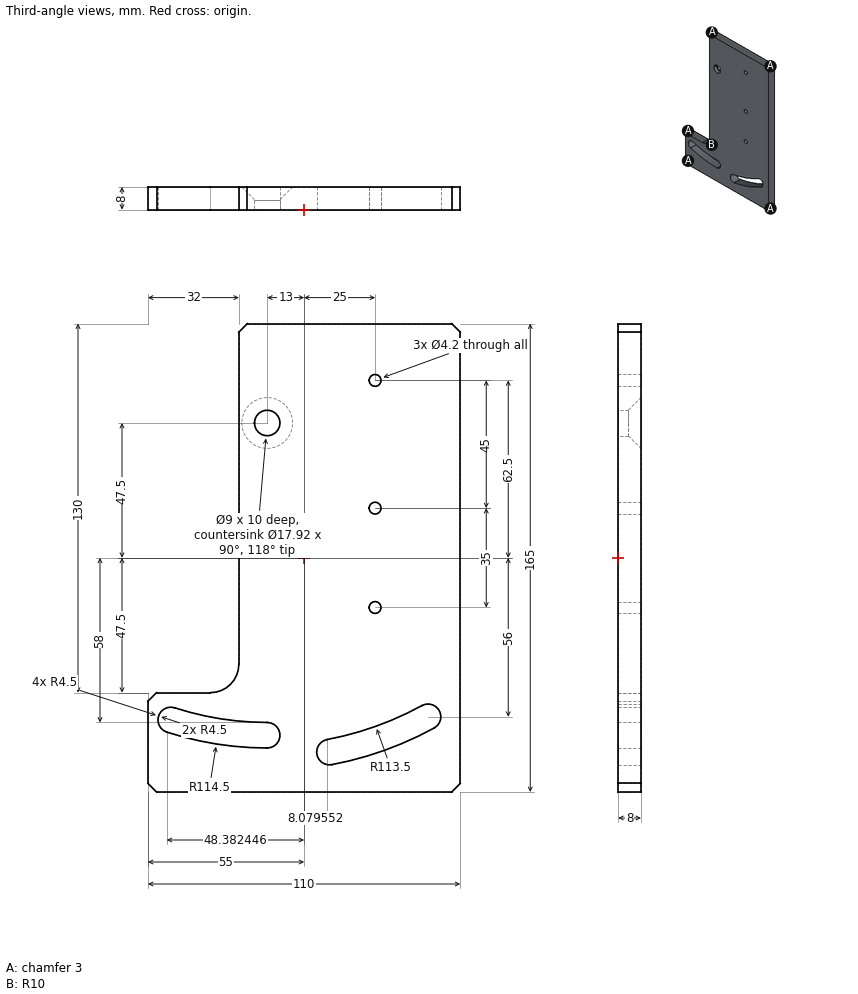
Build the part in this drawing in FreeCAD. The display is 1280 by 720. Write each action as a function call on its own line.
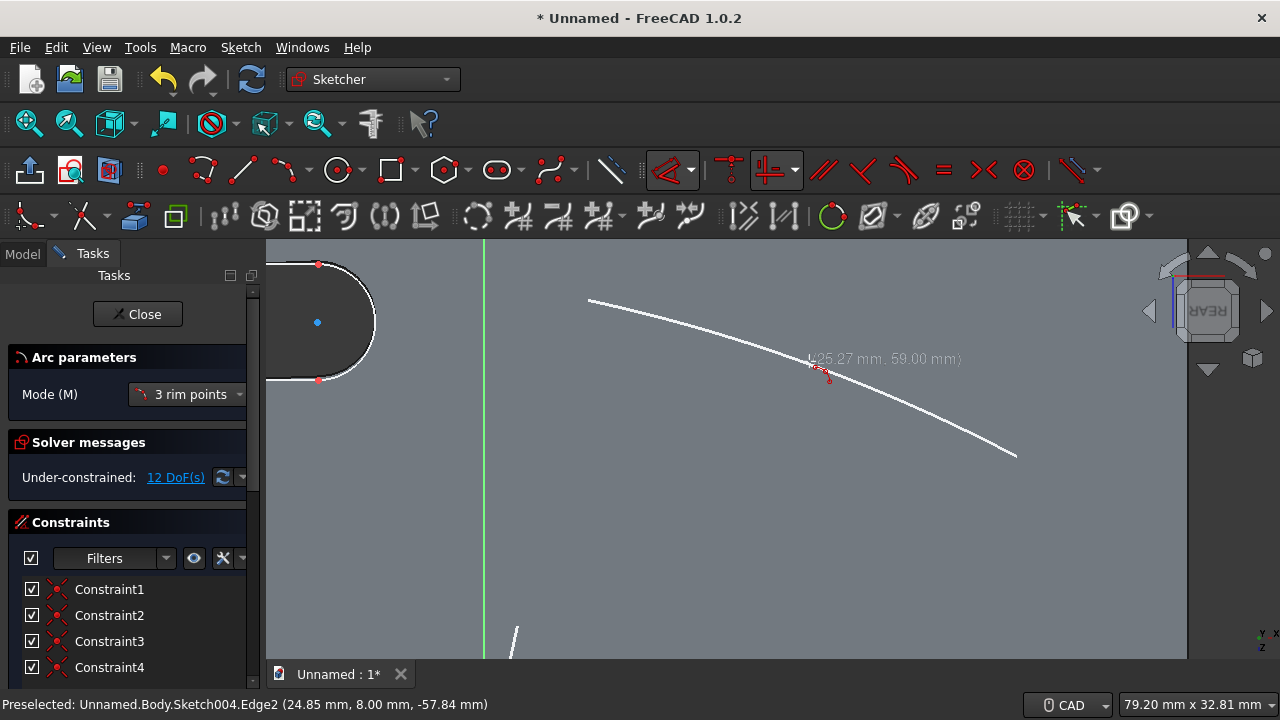
click(808, 359)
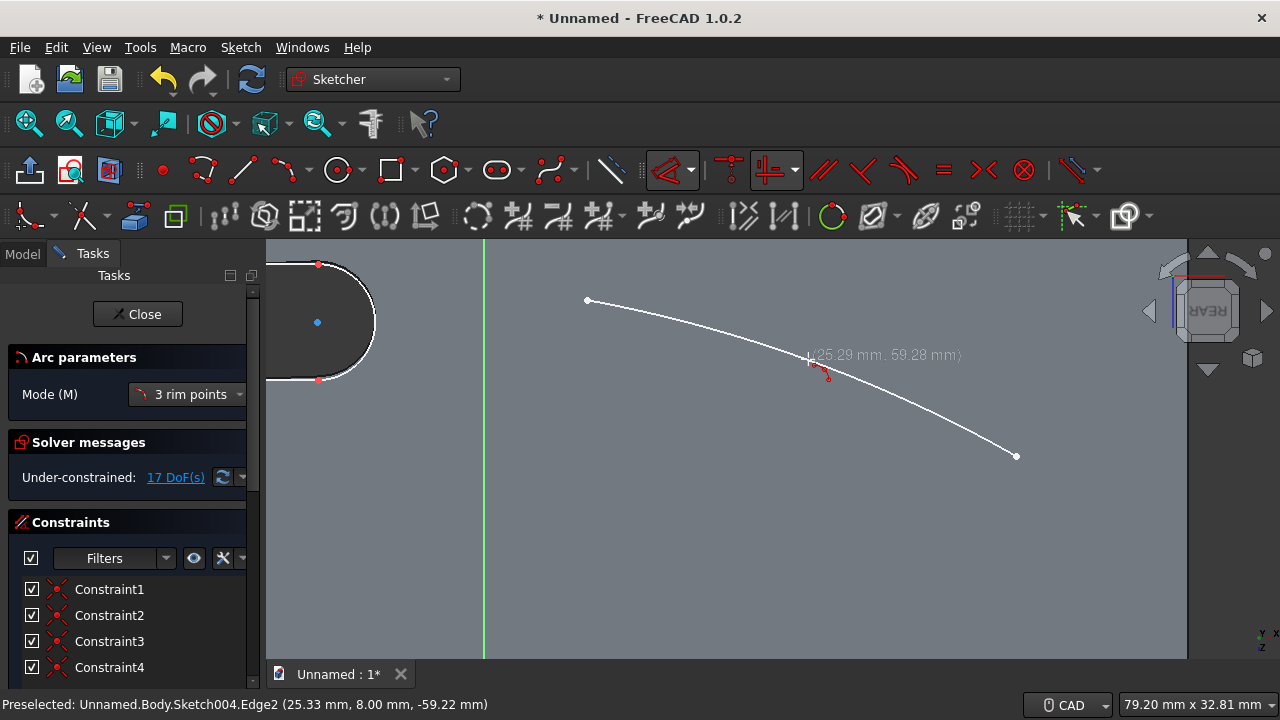
click(1017, 457)
click(1071, 352)
click(1094, 430)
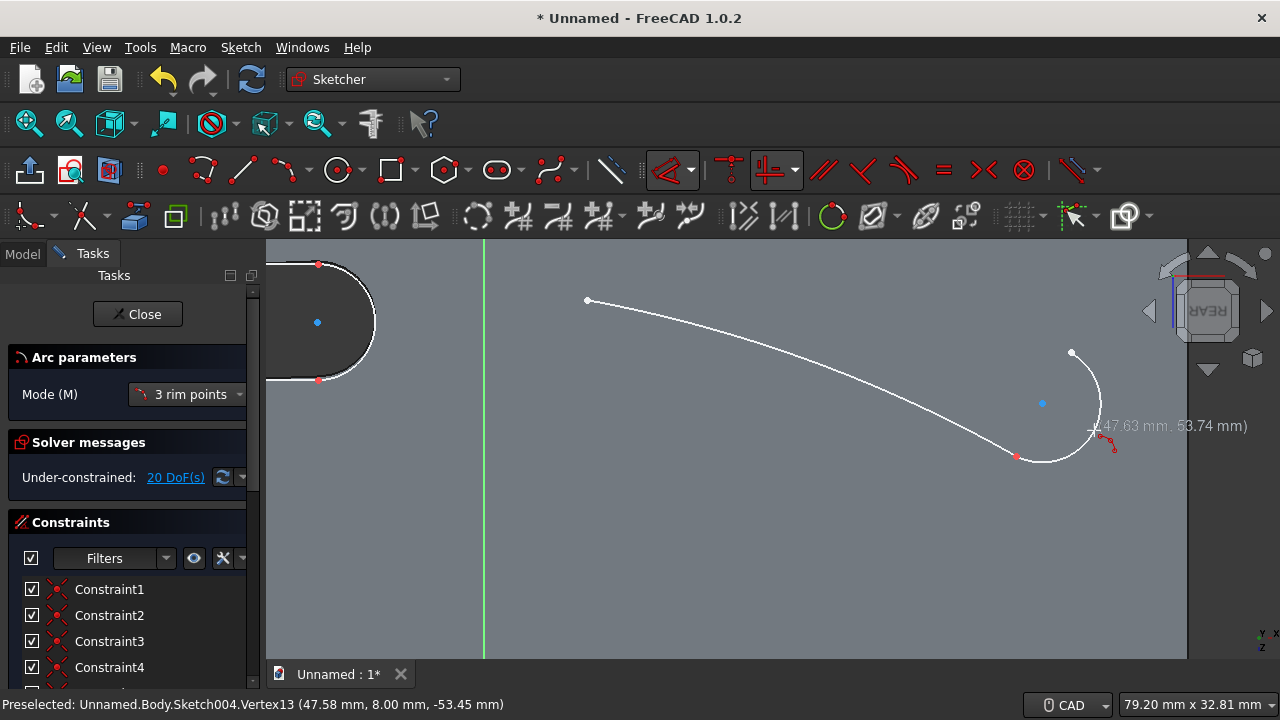
click(1071, 353)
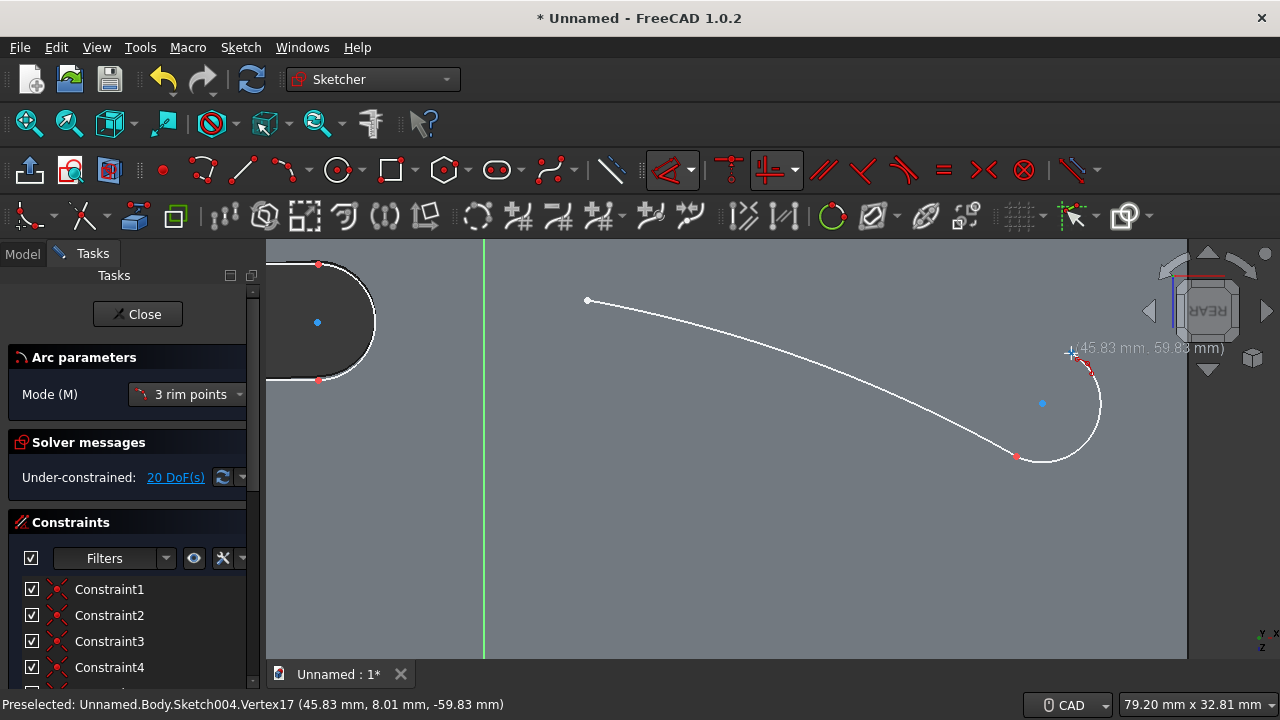
scroll(809, 361, down, 6)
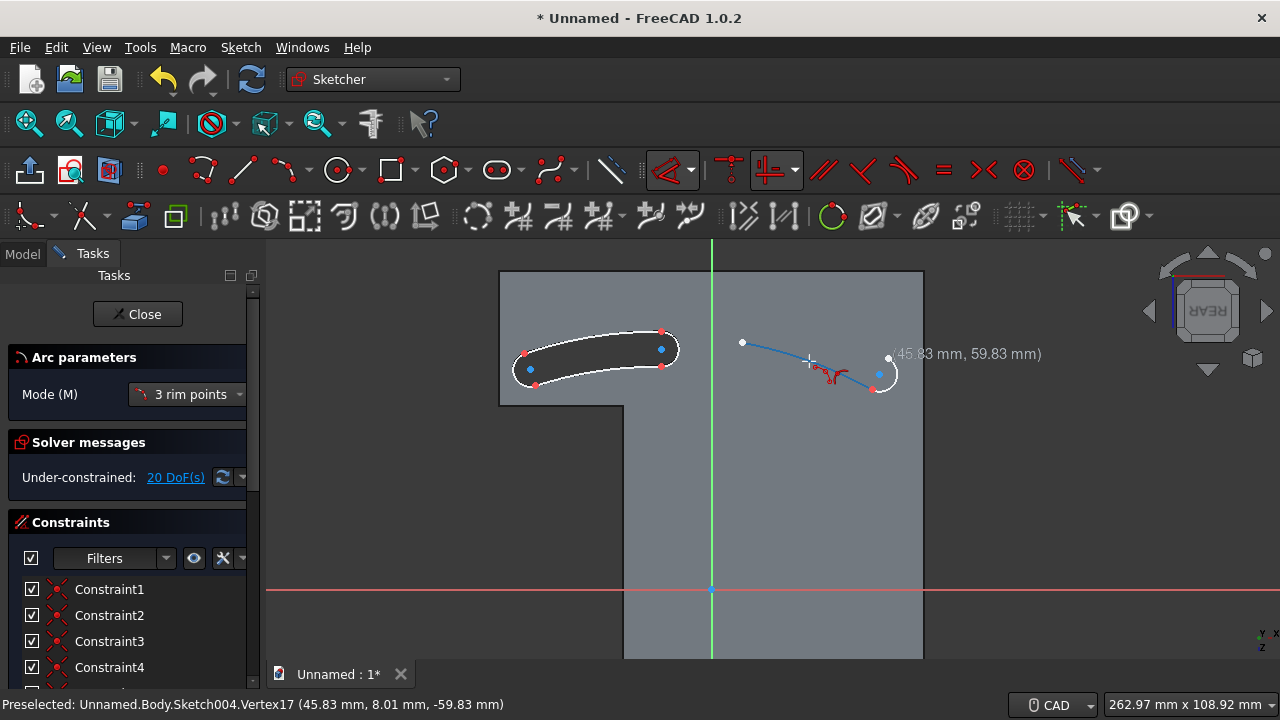
click(749, 309)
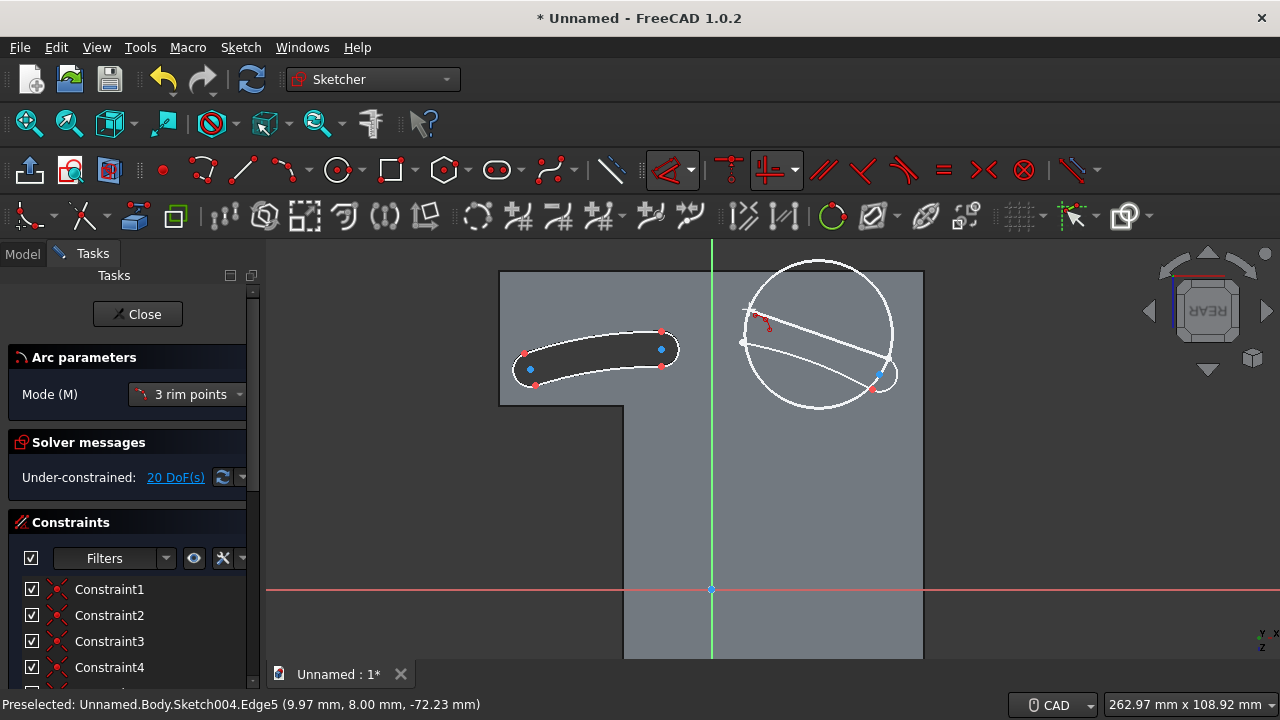
scroll(821, 328, up, 6)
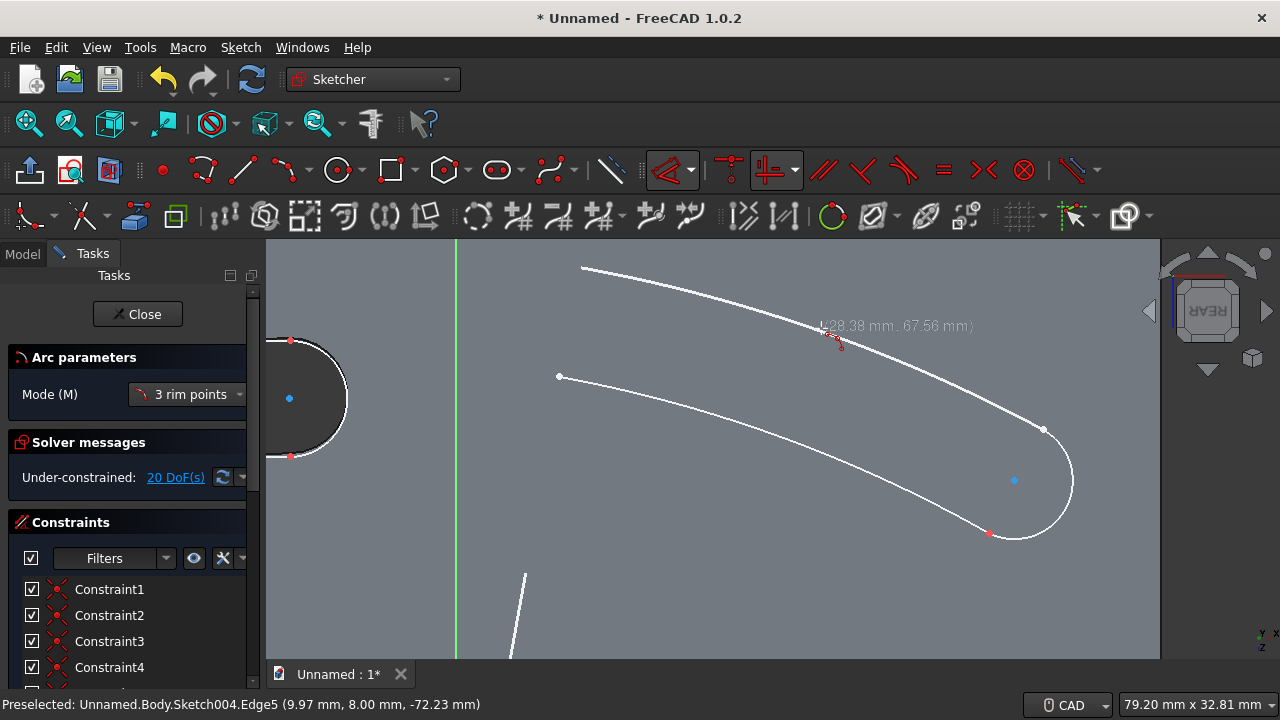
click(819, 327)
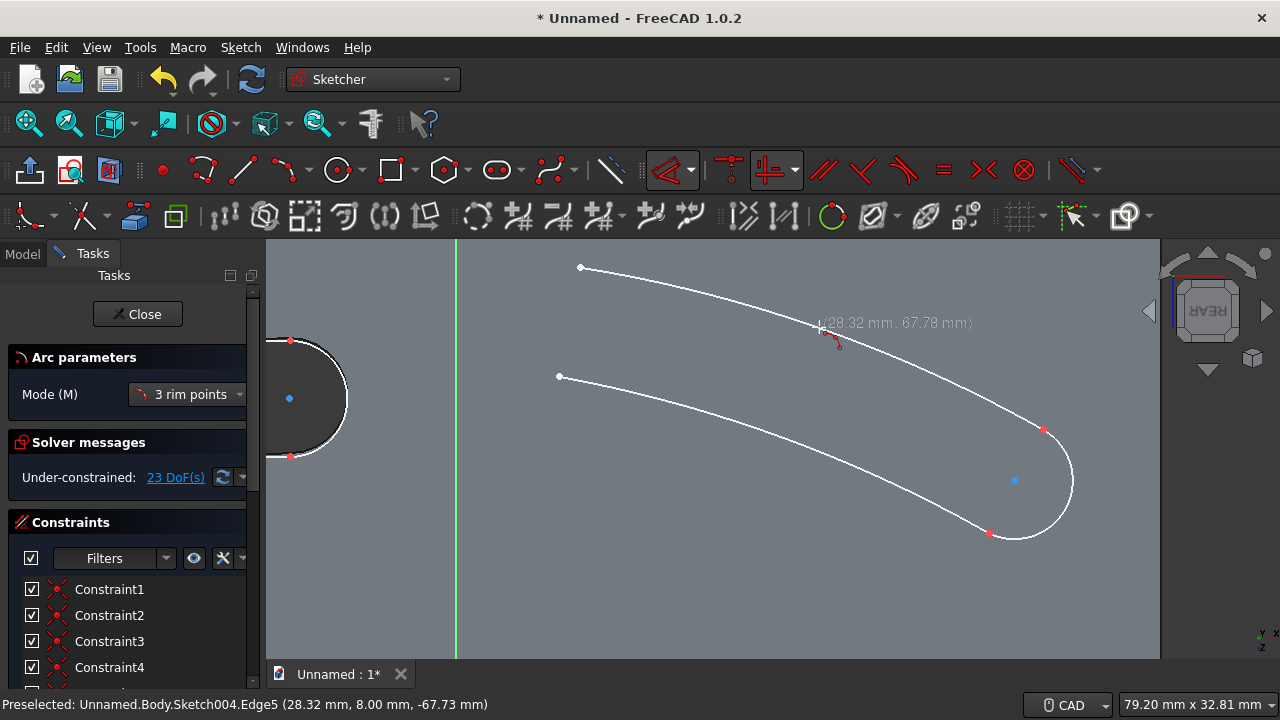
scroll(822, 328, down, 6)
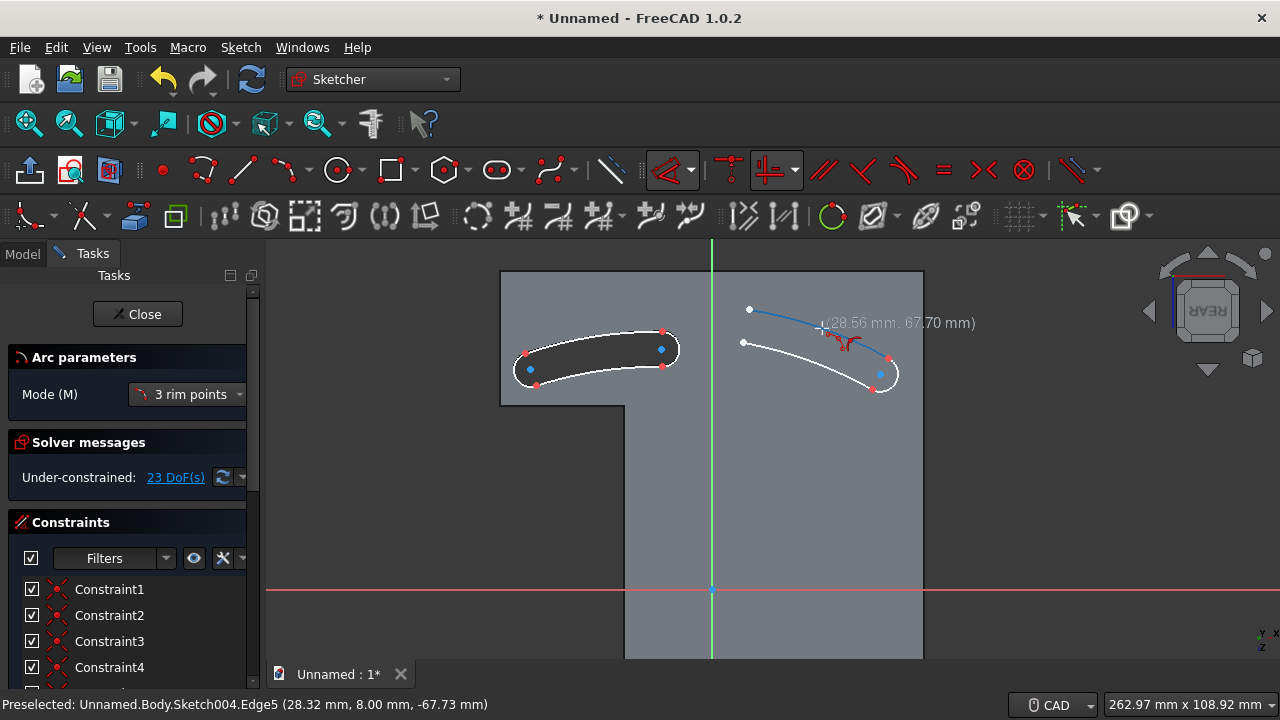
click(750, 310)
click(743, 343)
click(730, 322)
key(Escape)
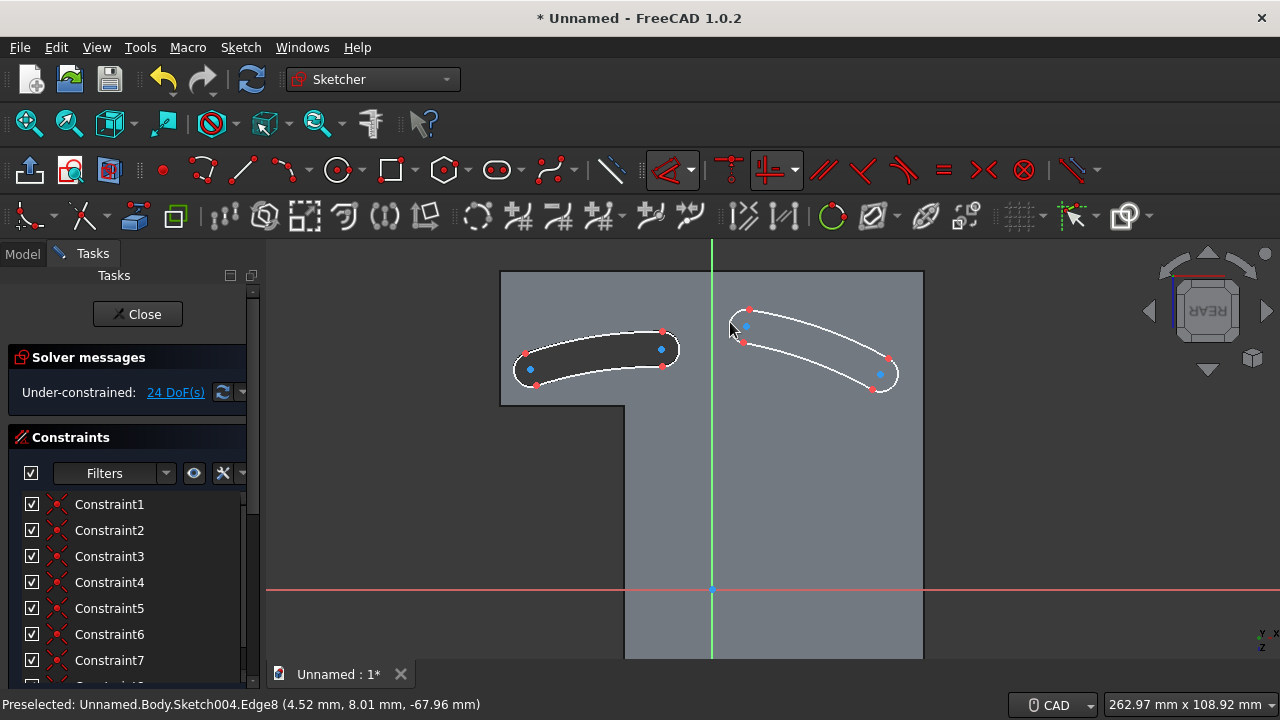
click(676, 360)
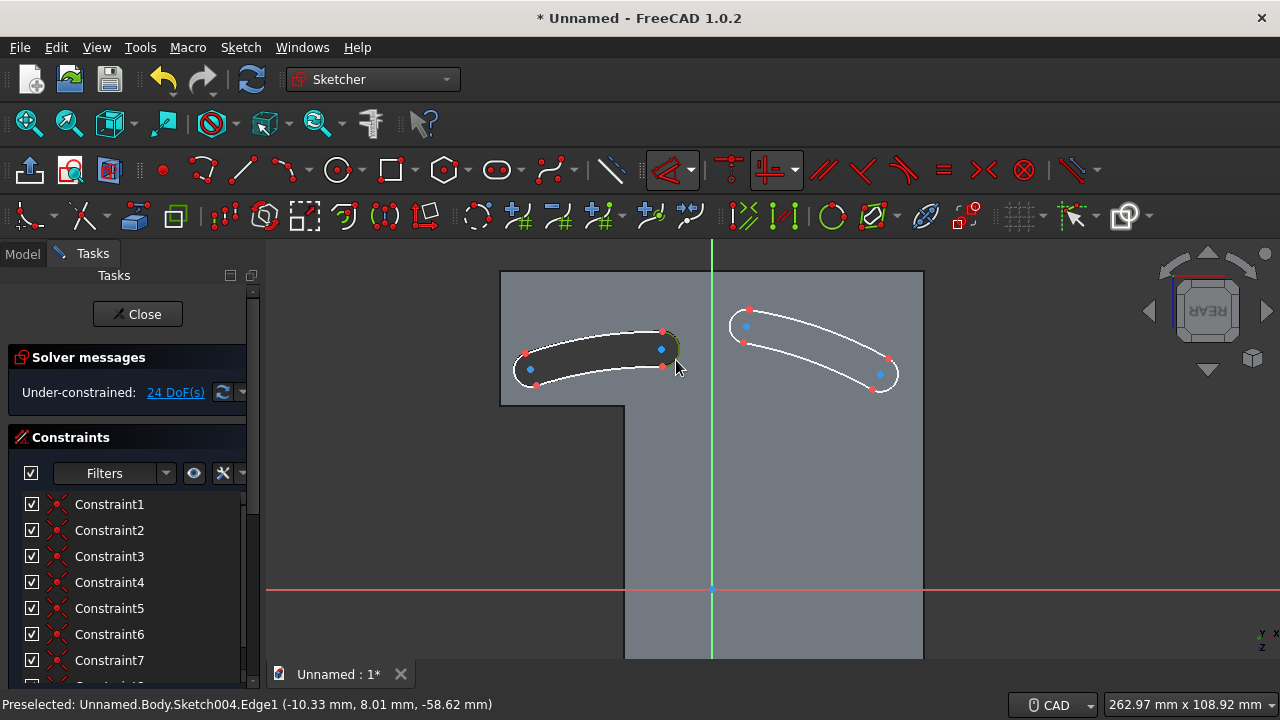
click(621, 333)